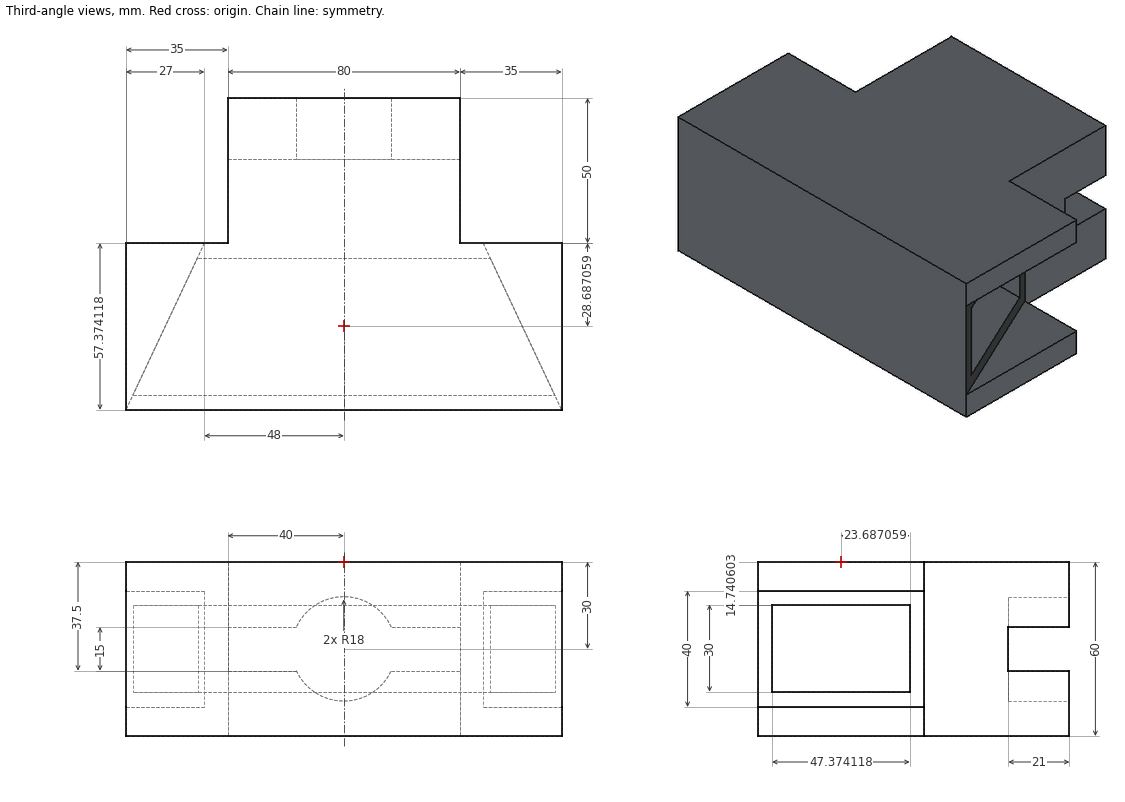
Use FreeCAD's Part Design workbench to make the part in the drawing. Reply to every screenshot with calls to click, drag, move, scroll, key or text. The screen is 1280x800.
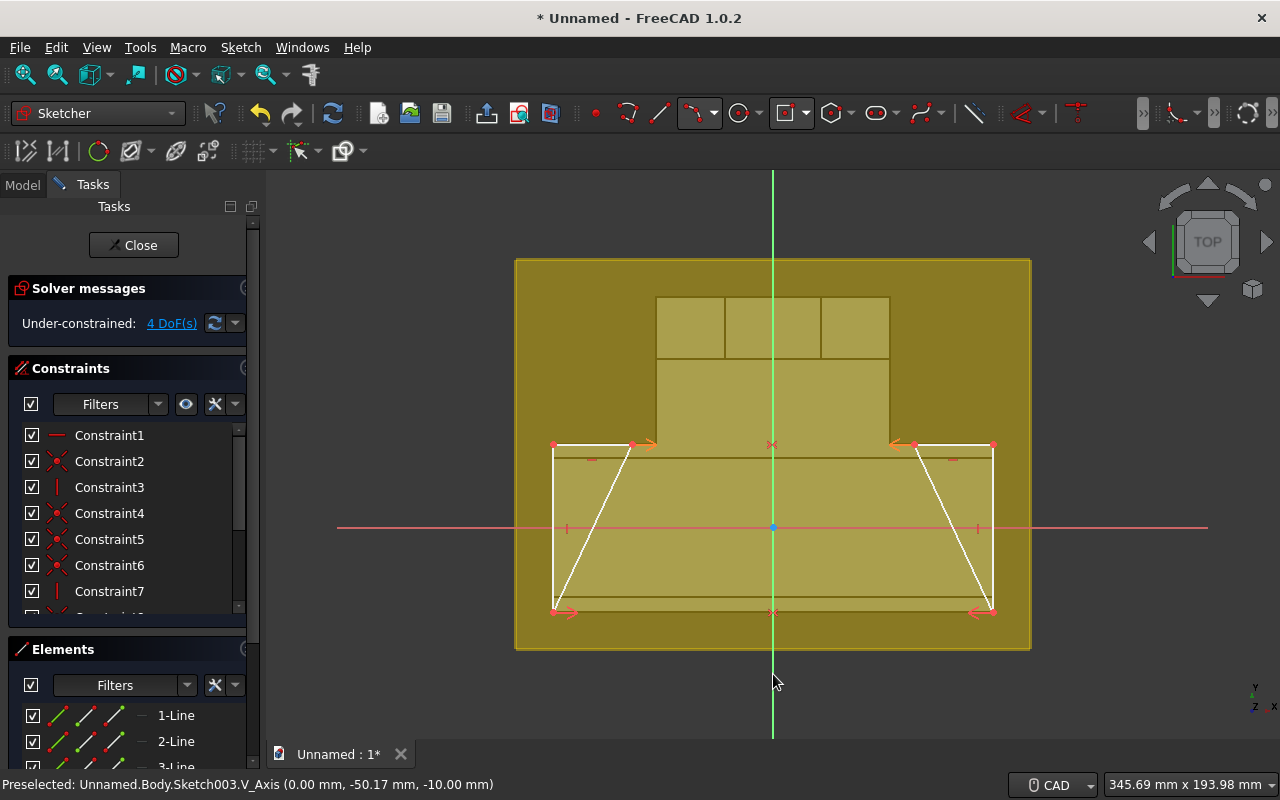
click(608, 445)
click(593, 411)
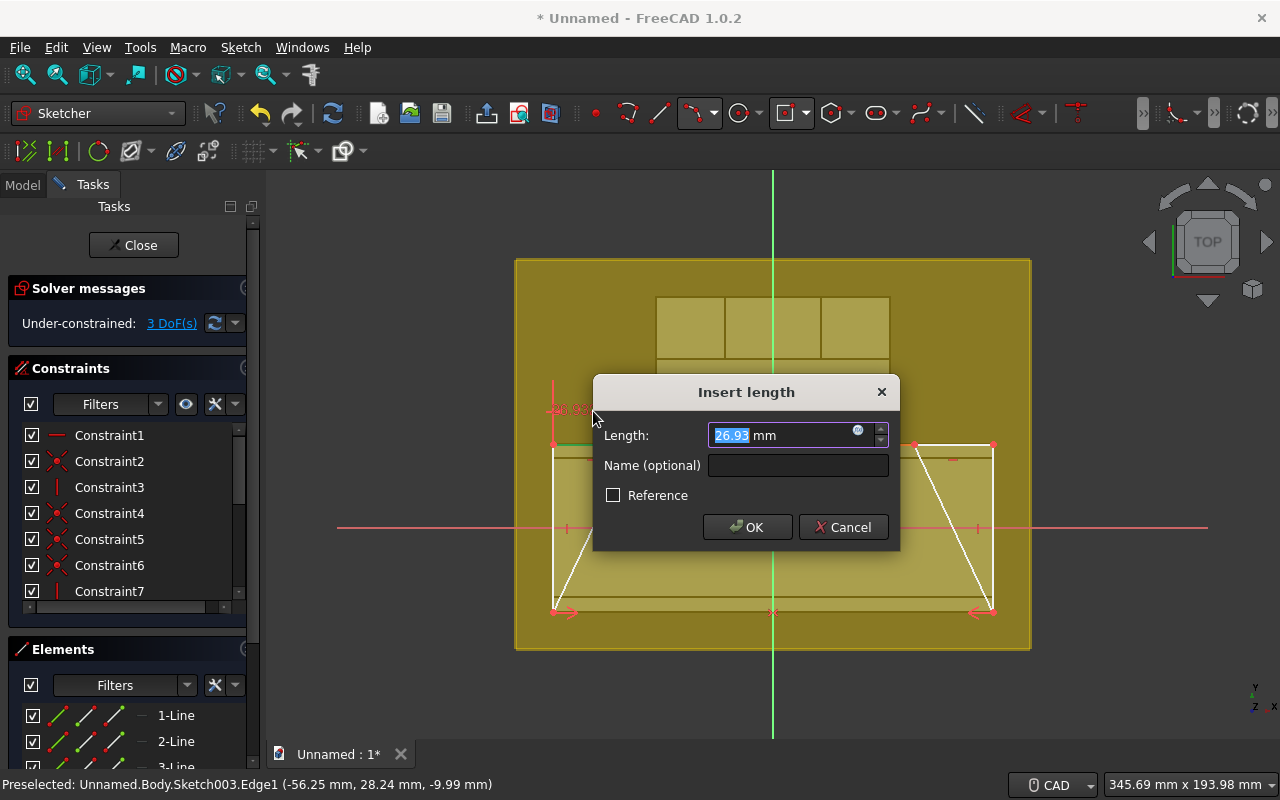
text(27)
key(Return)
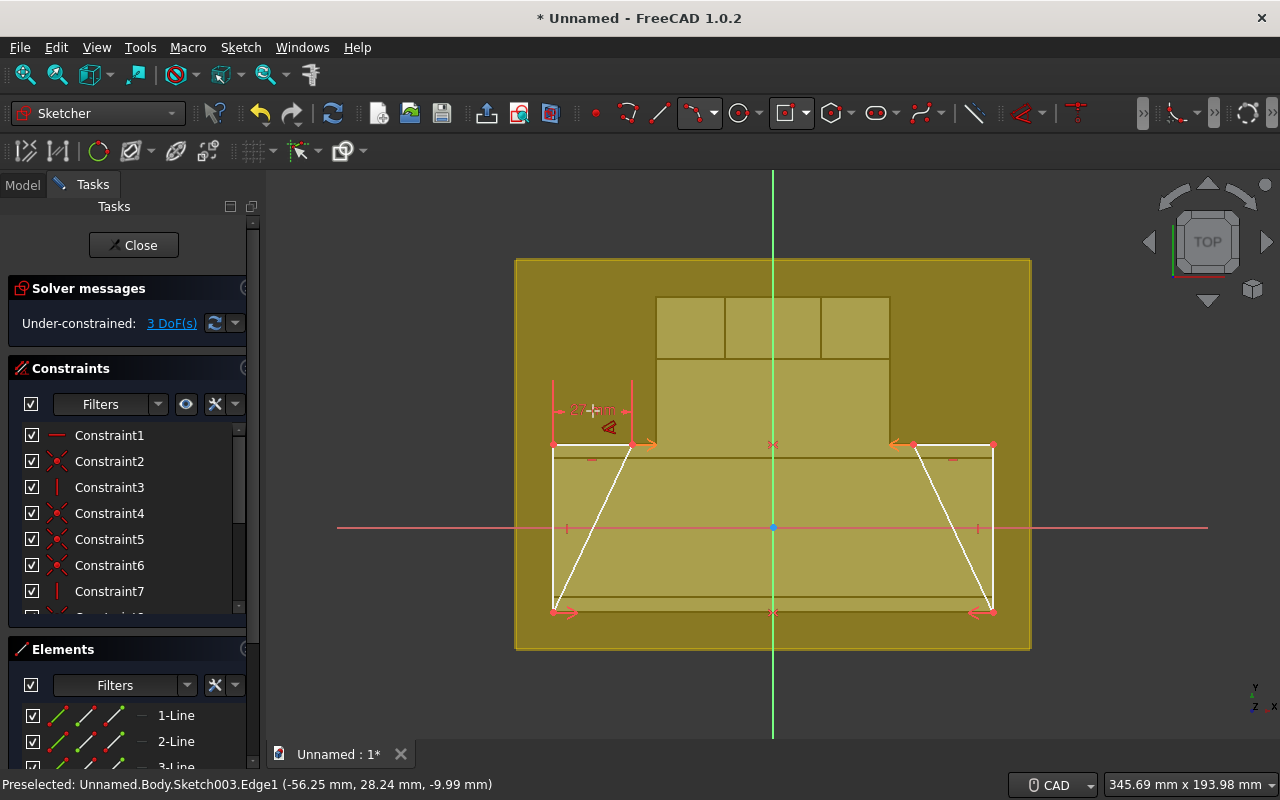
click(632, 445)
click(703, 411)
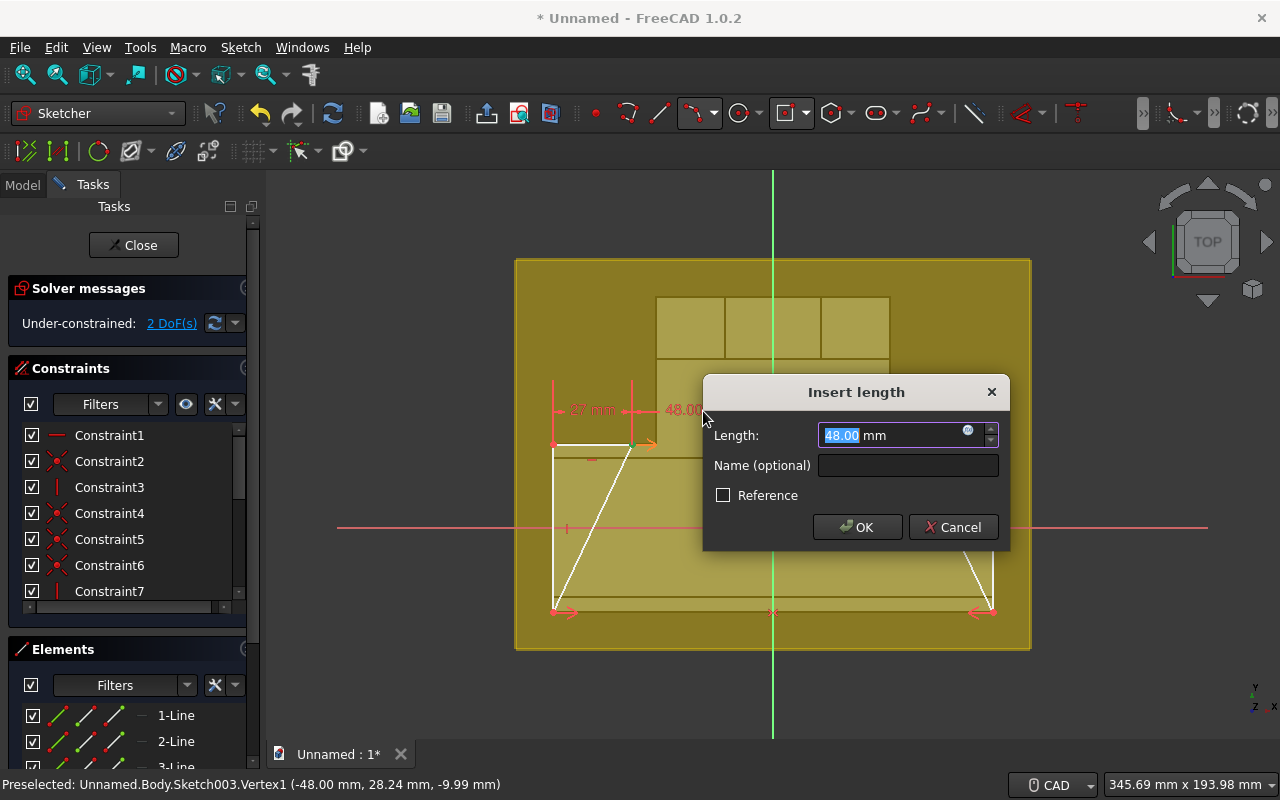
text(48)
key(Return)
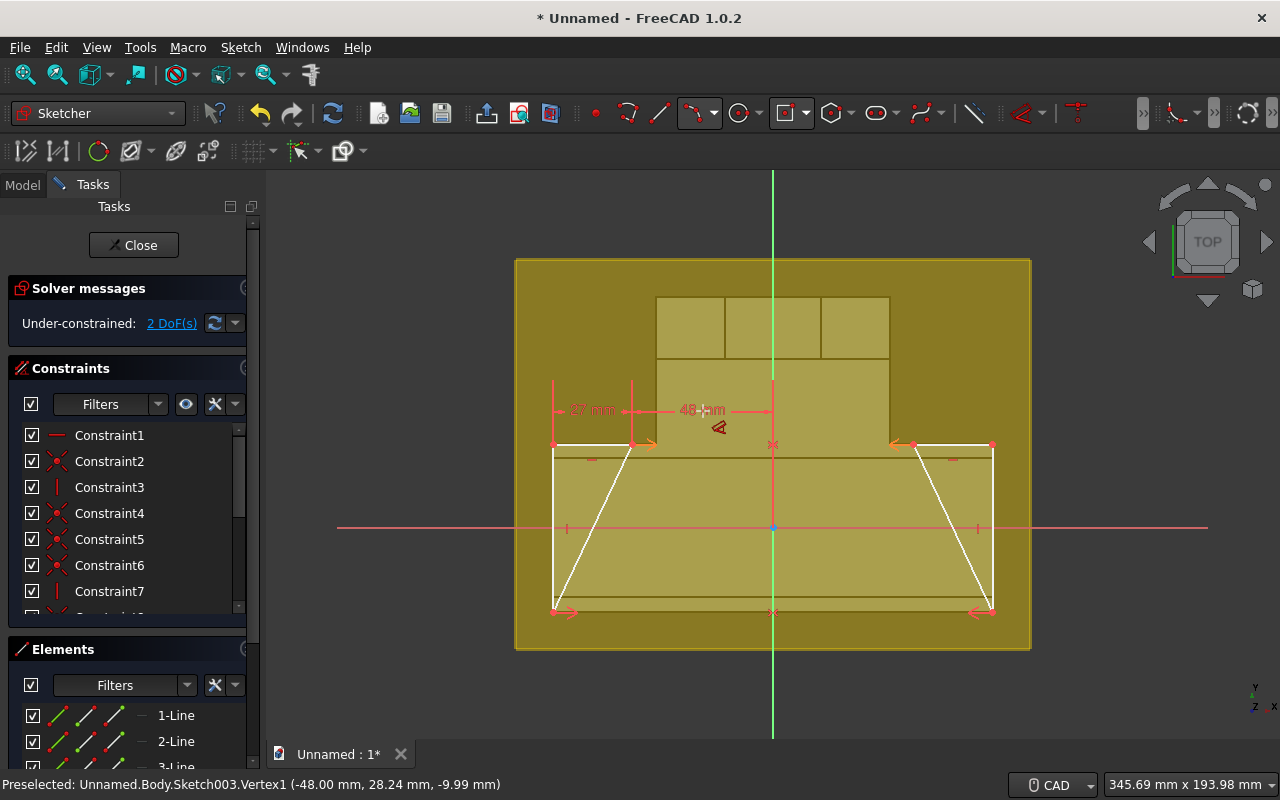
click(553, 495)
click(519, 490)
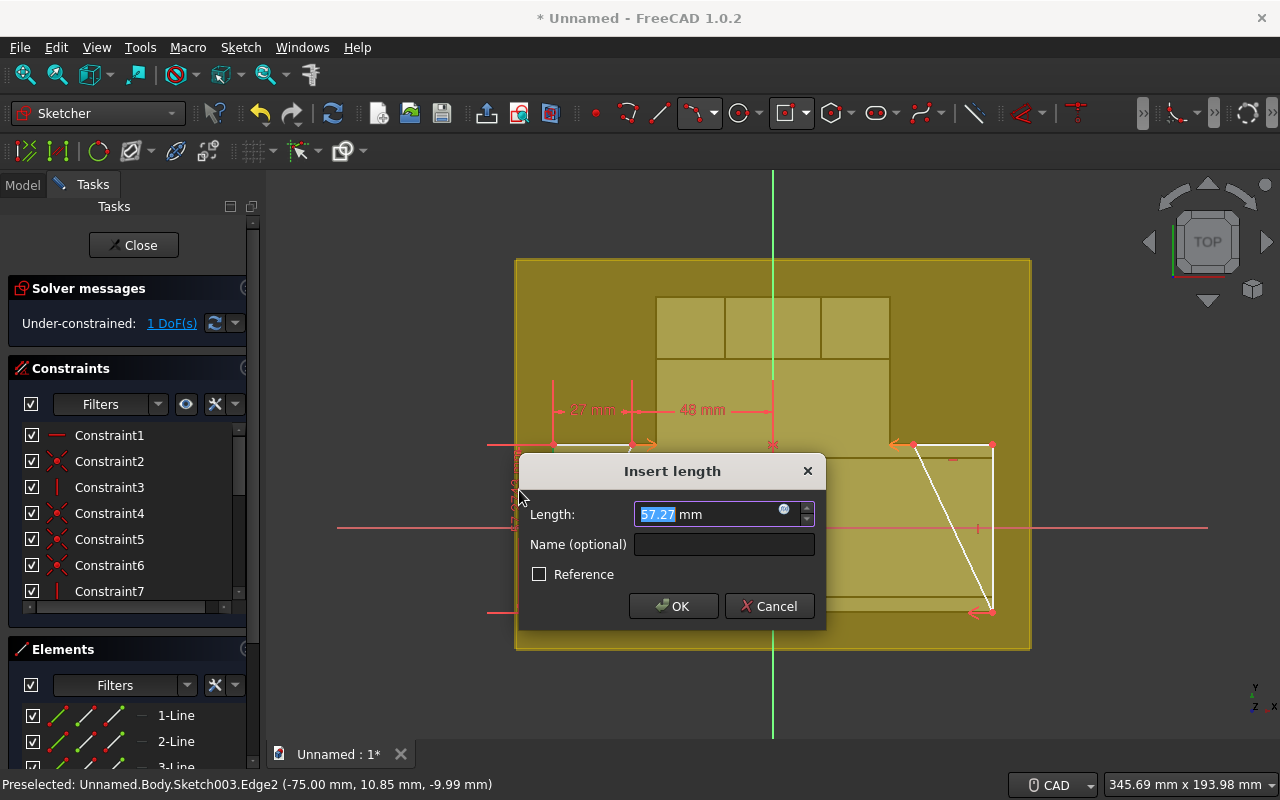
text(57.374118)
key(Return)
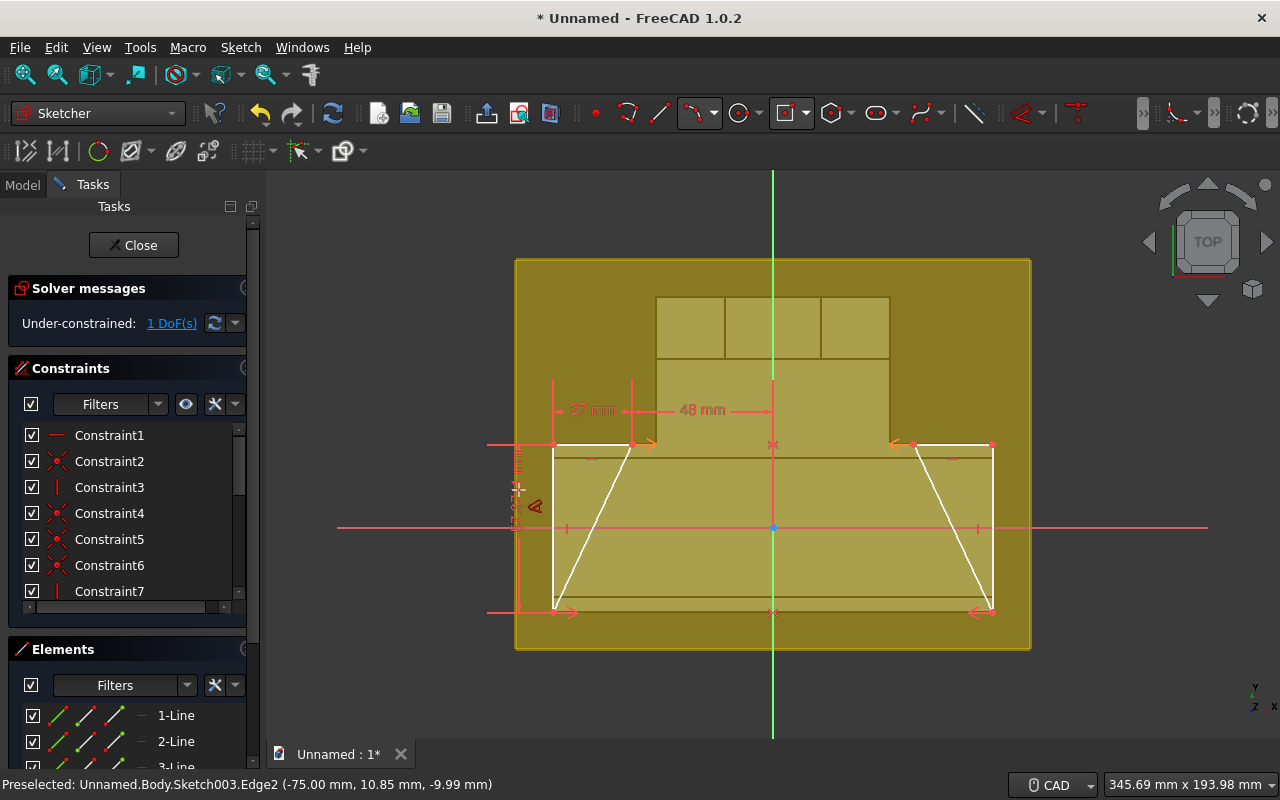
click(632, 445)
click(598, 486)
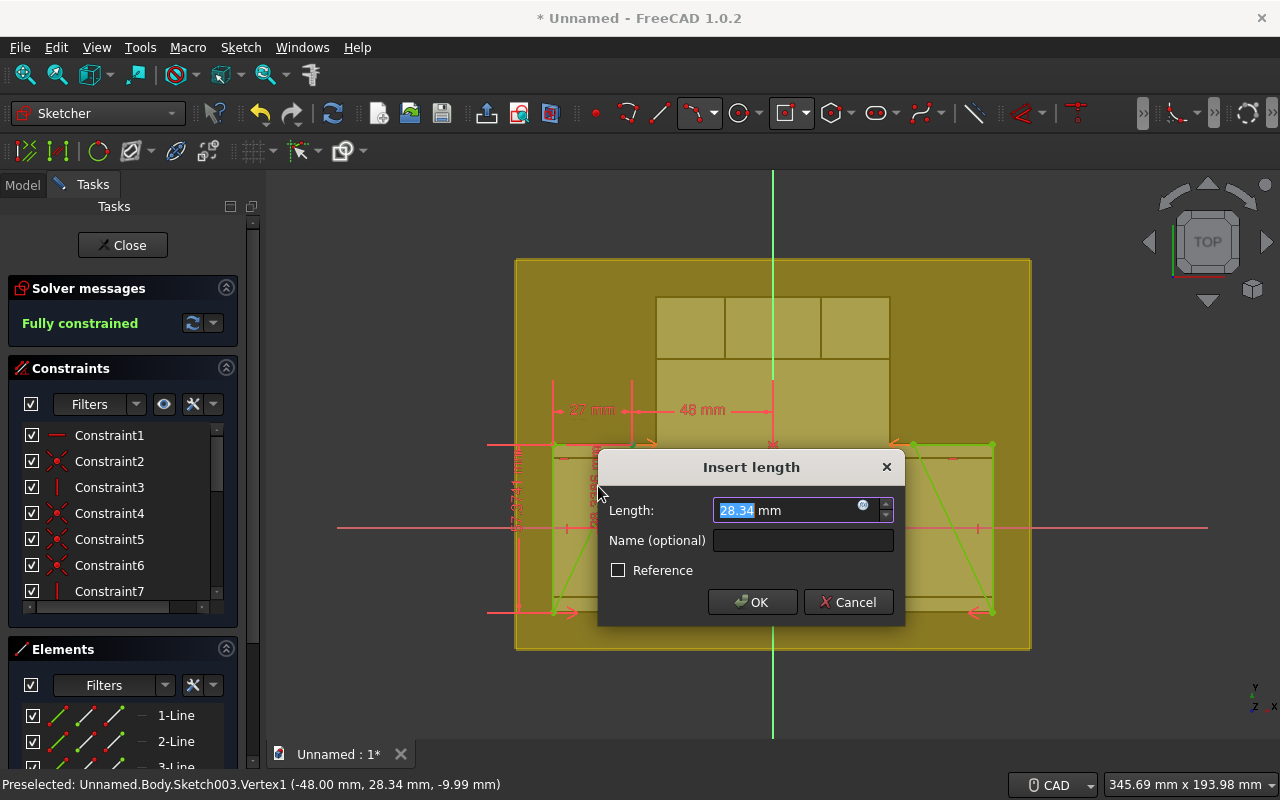
text(28.687059)
key(Return)
key(Escape)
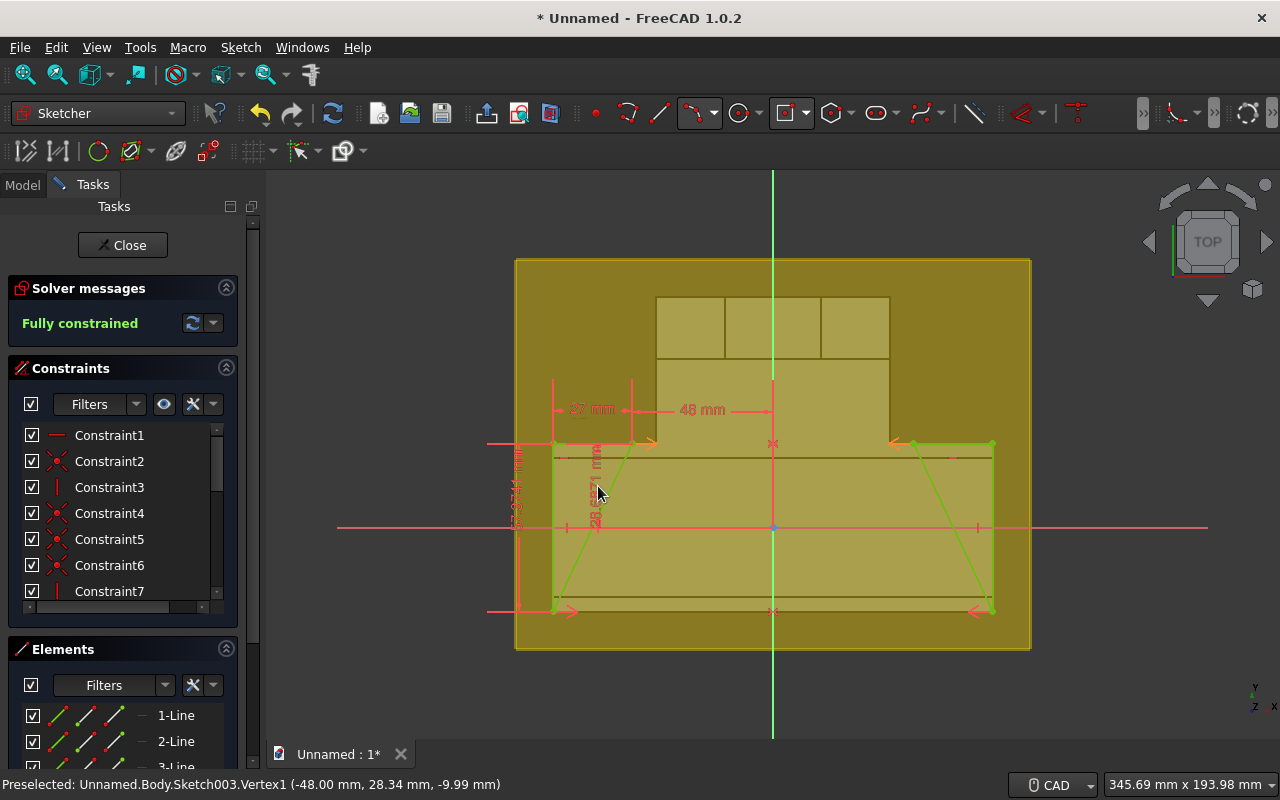
click(123, 245)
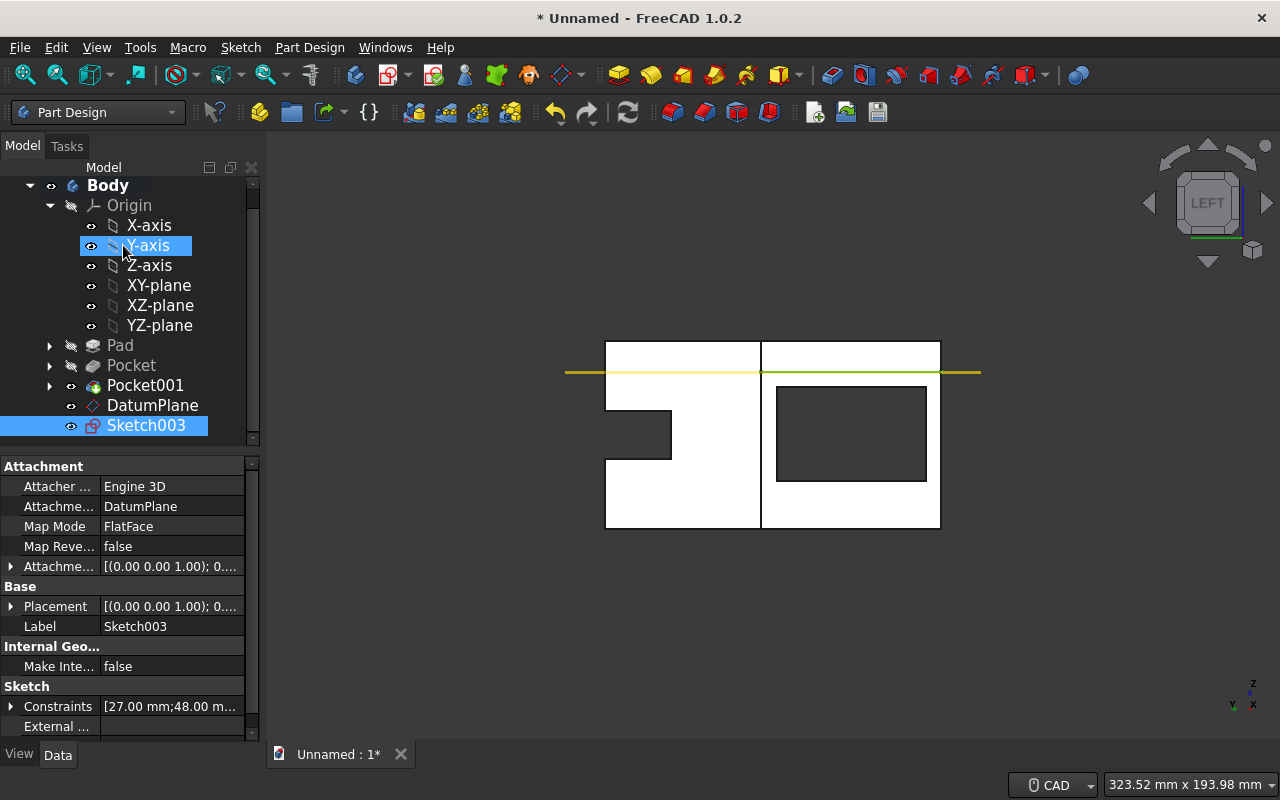
click(834, 76)